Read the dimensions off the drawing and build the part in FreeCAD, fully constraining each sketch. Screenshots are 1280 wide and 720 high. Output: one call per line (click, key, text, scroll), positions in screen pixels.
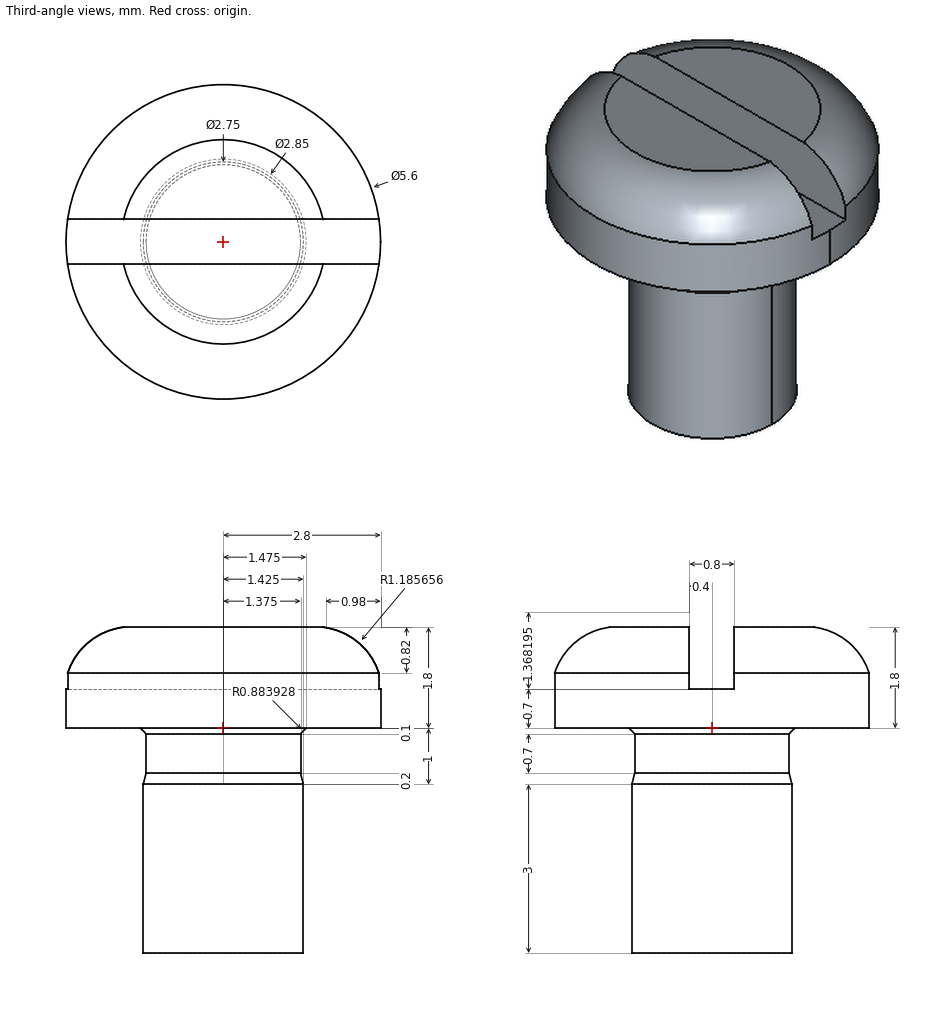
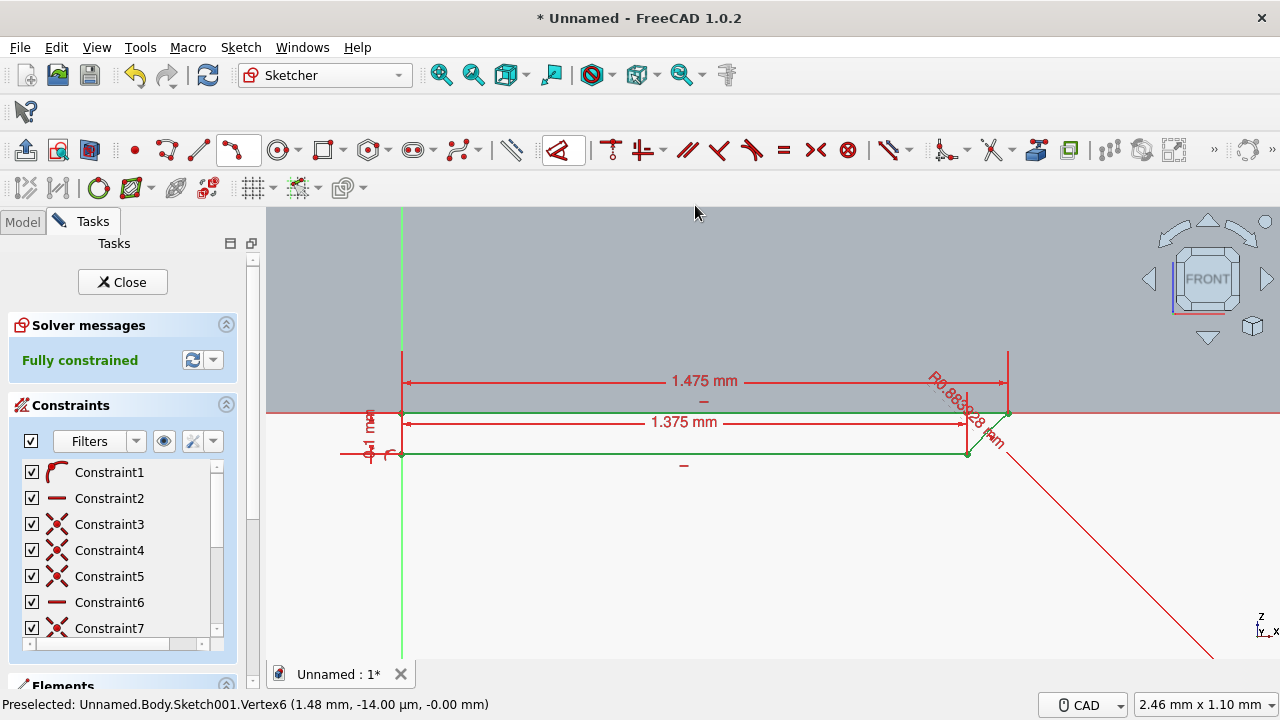
click(123, 282)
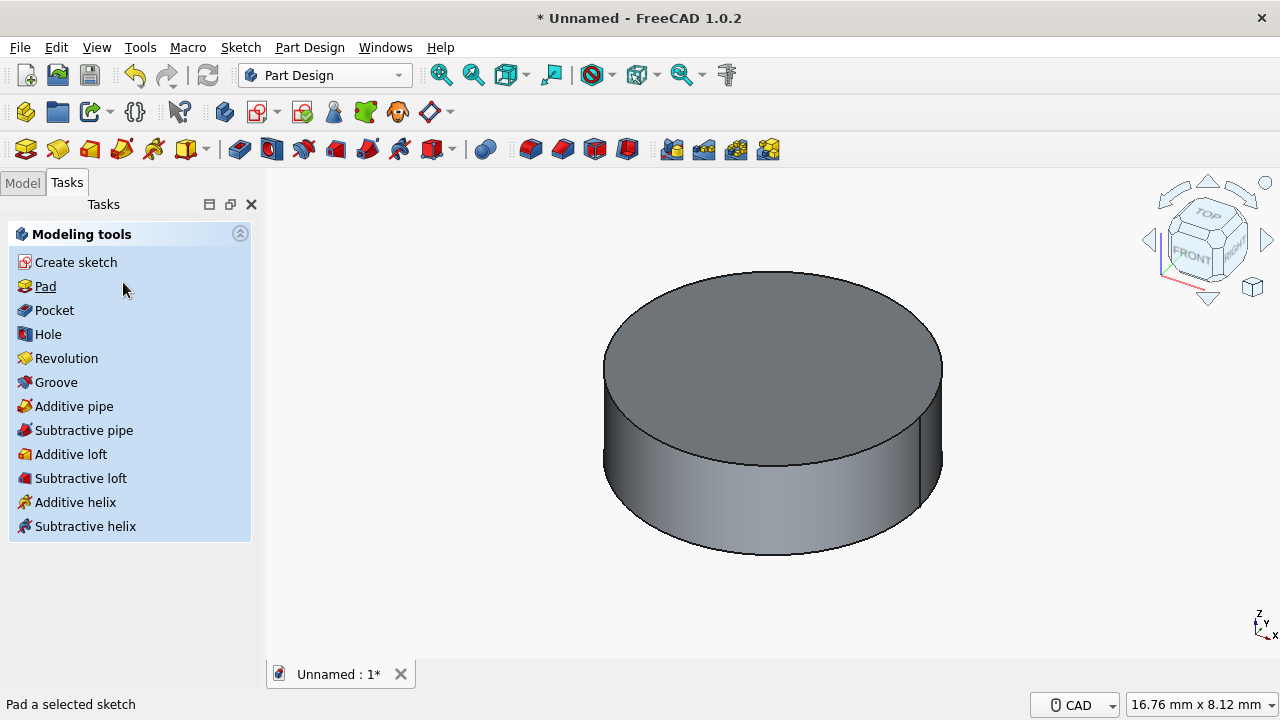
click(58, 150)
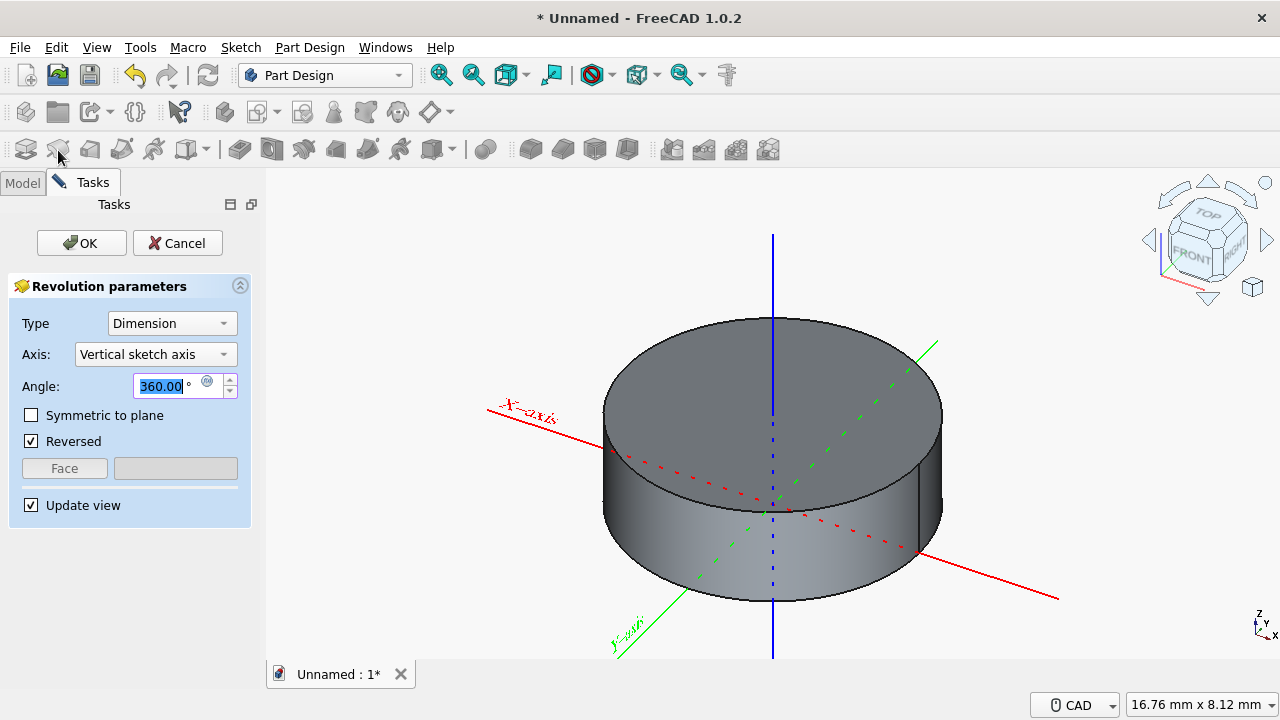
click(82, 243)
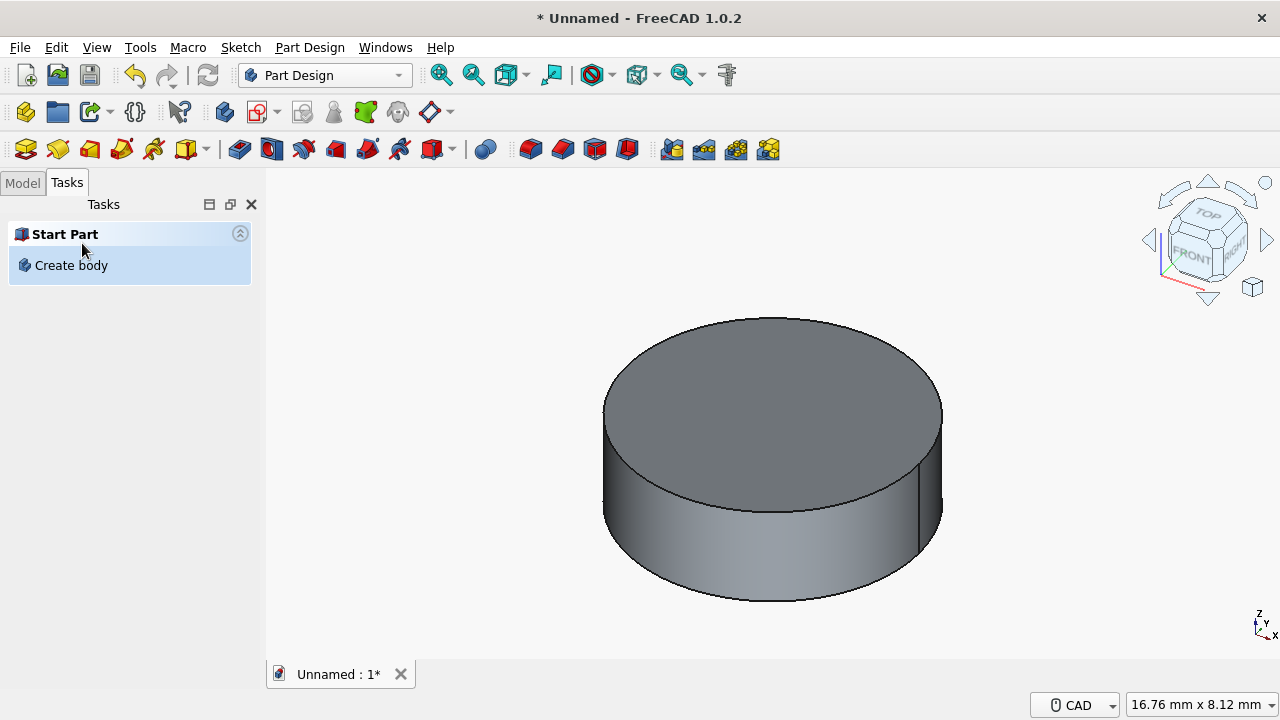
key(5)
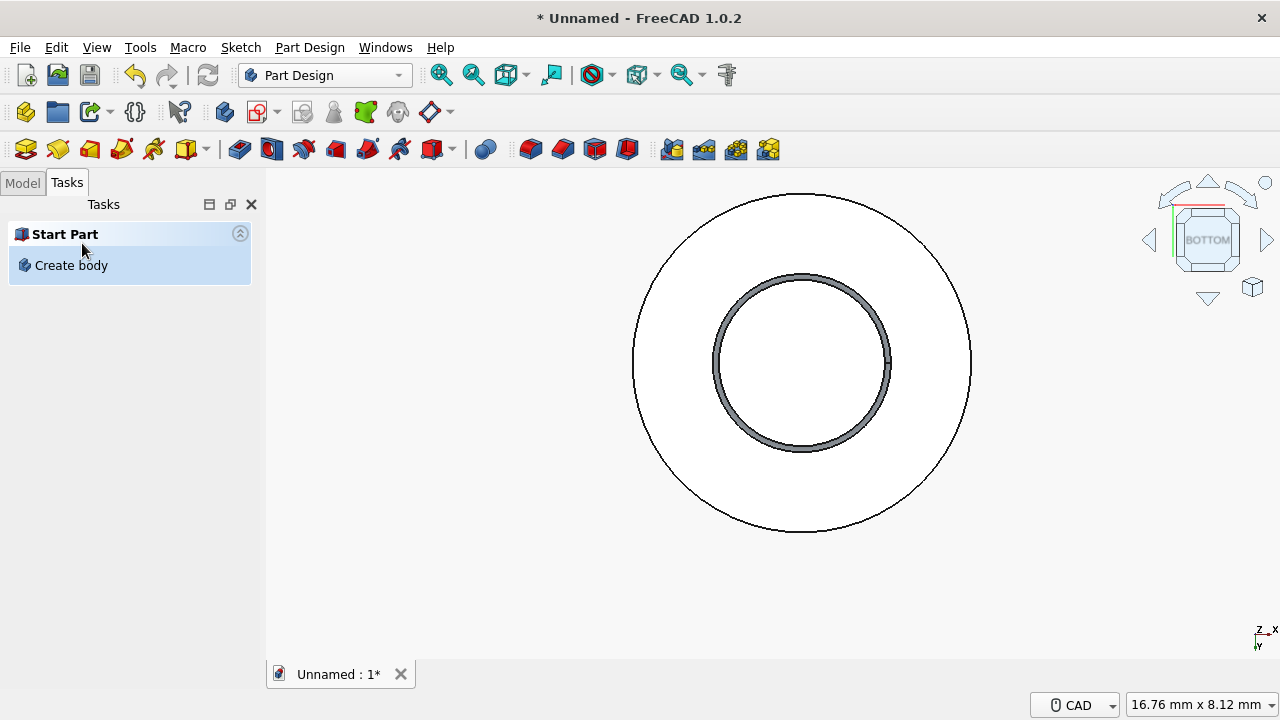
click(802, 362)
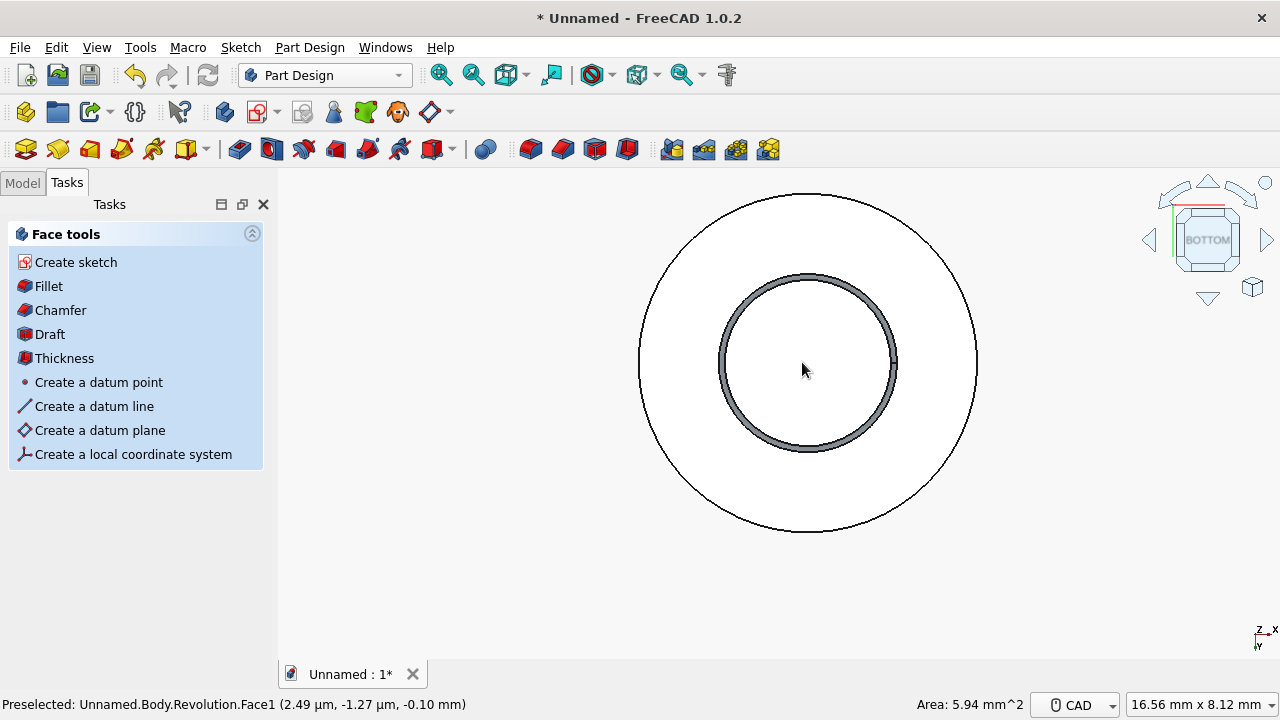
click(258, 112)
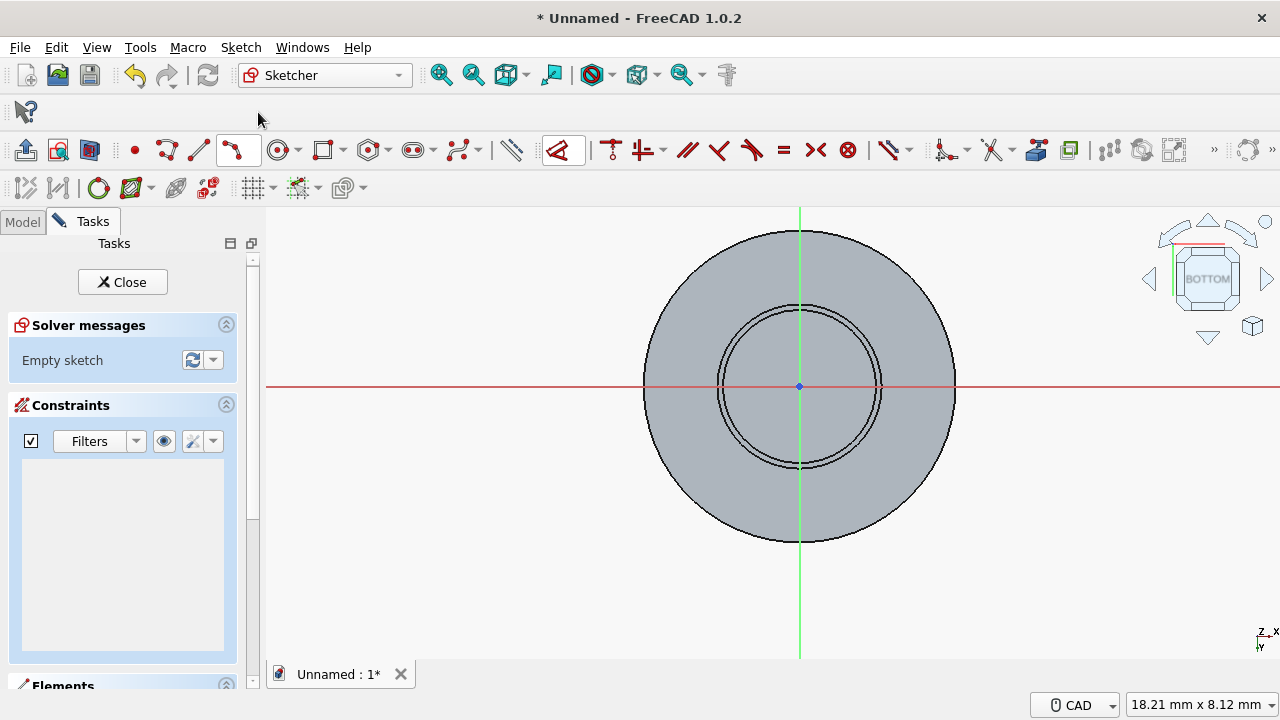
scroll(915, 330, up, 3)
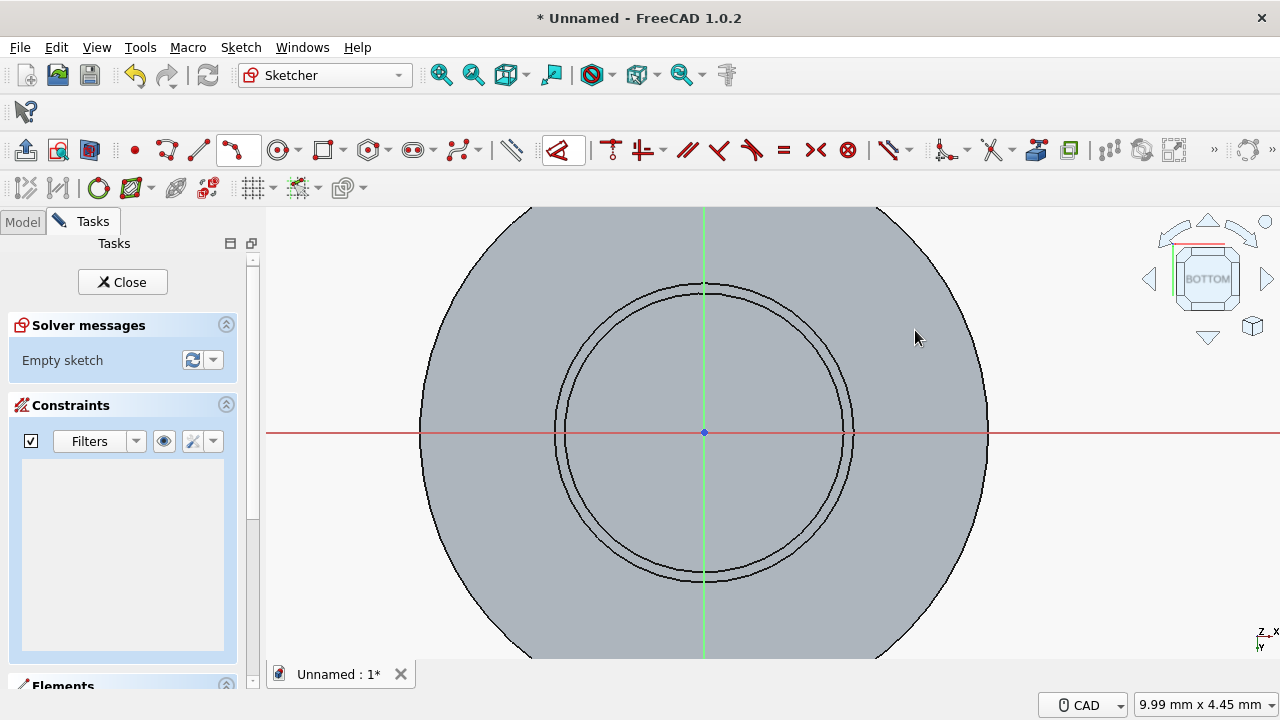
click(278, 150)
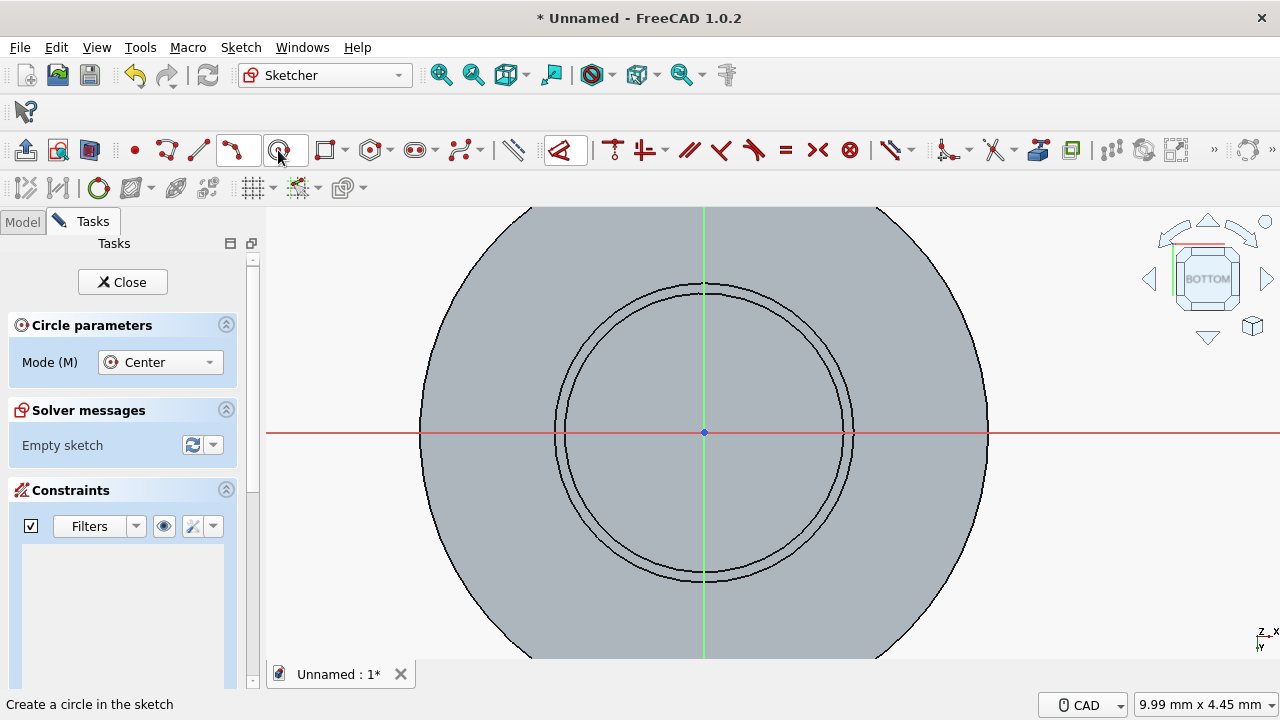
click(704, 433)
click(803, 334)
key(Escape)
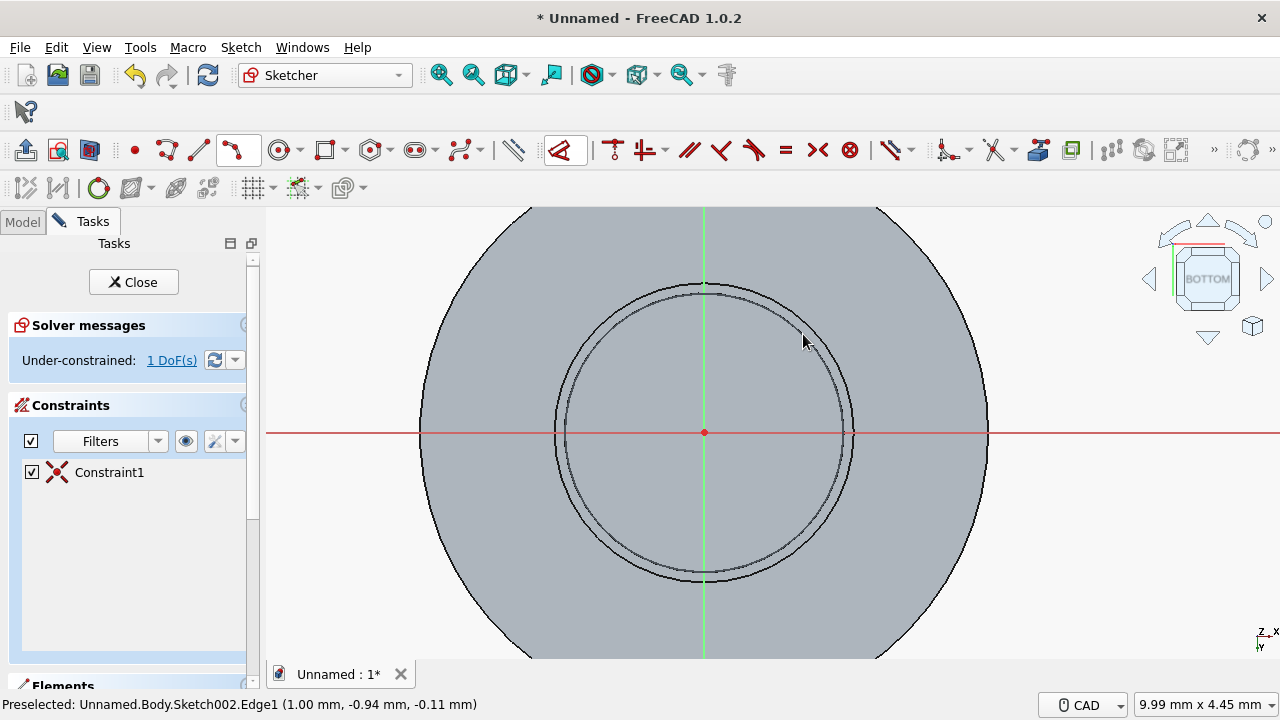
click(802, 334)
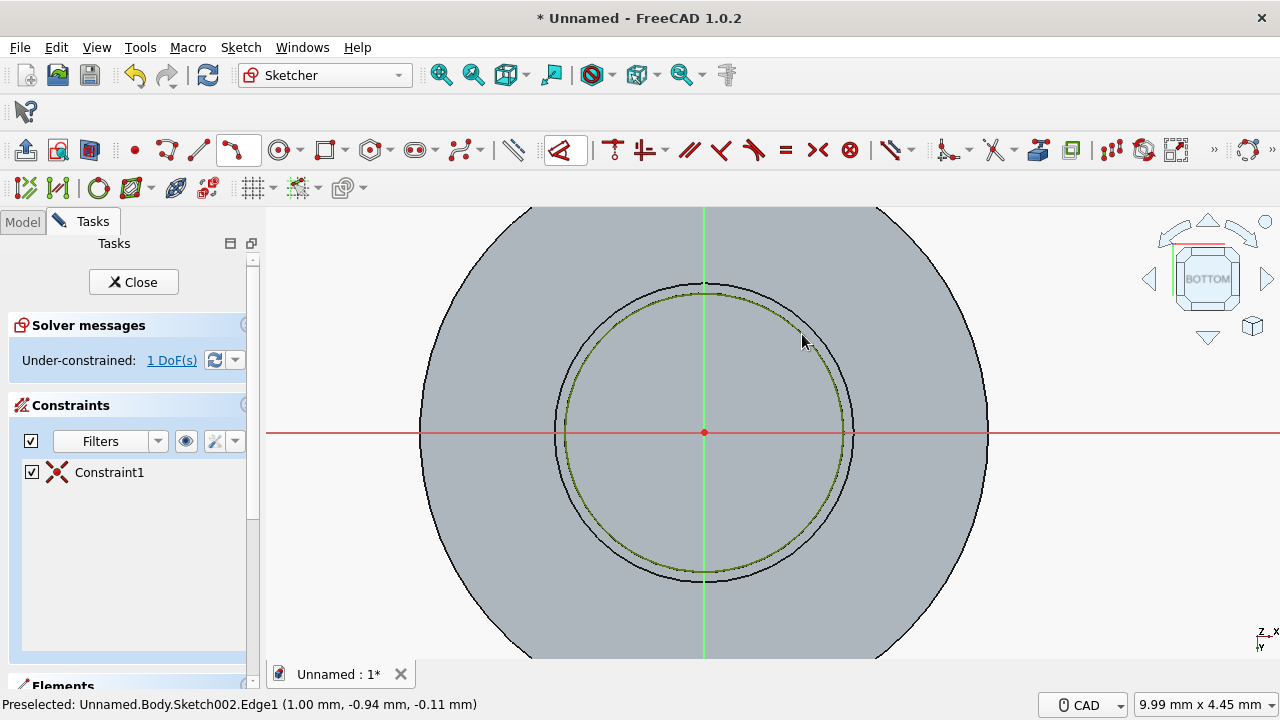
click(582, 150)